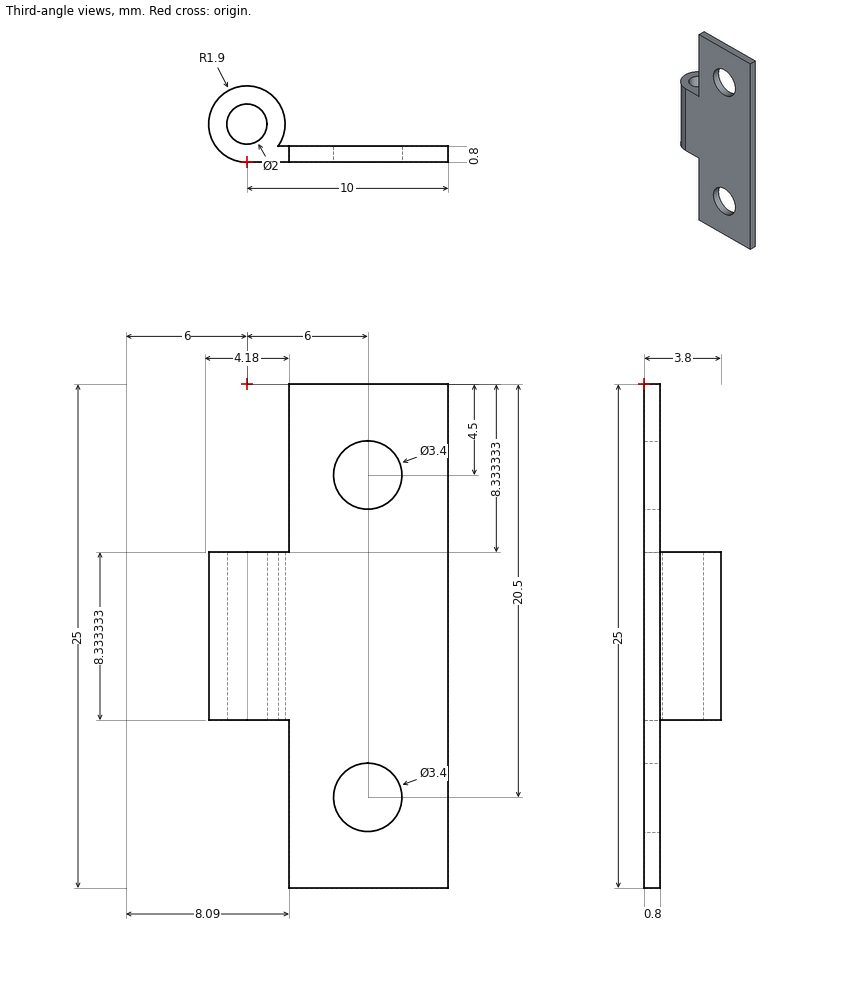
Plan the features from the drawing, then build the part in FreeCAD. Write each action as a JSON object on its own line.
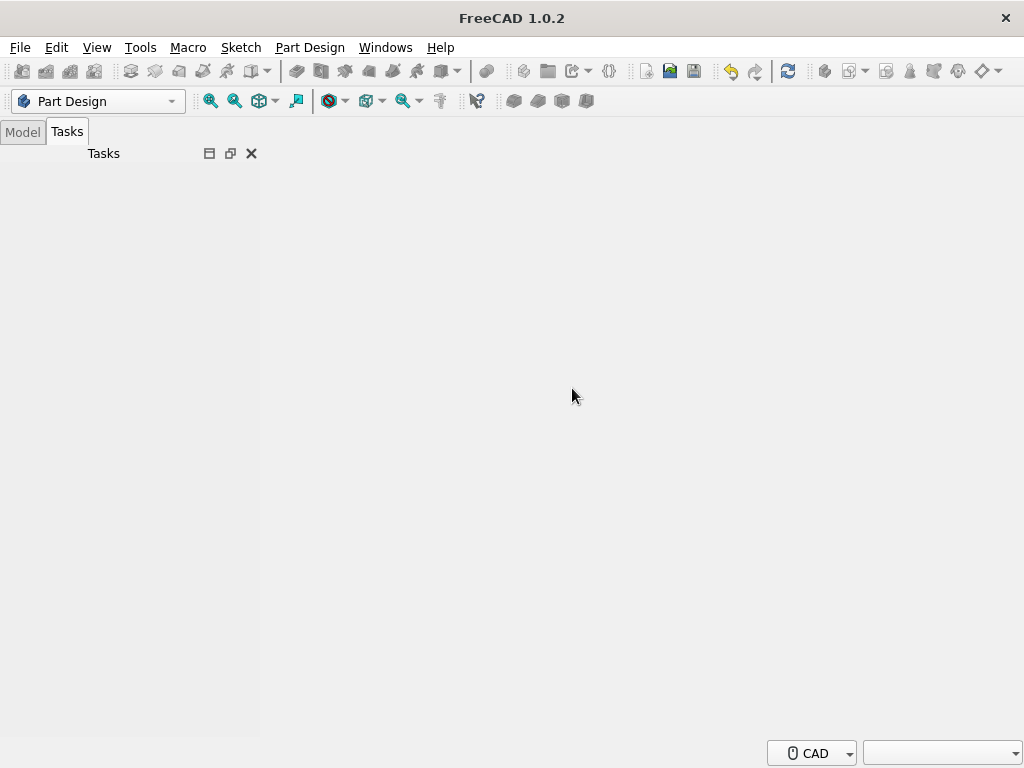
{"action": "left_click", "coordinate": [646, 72]}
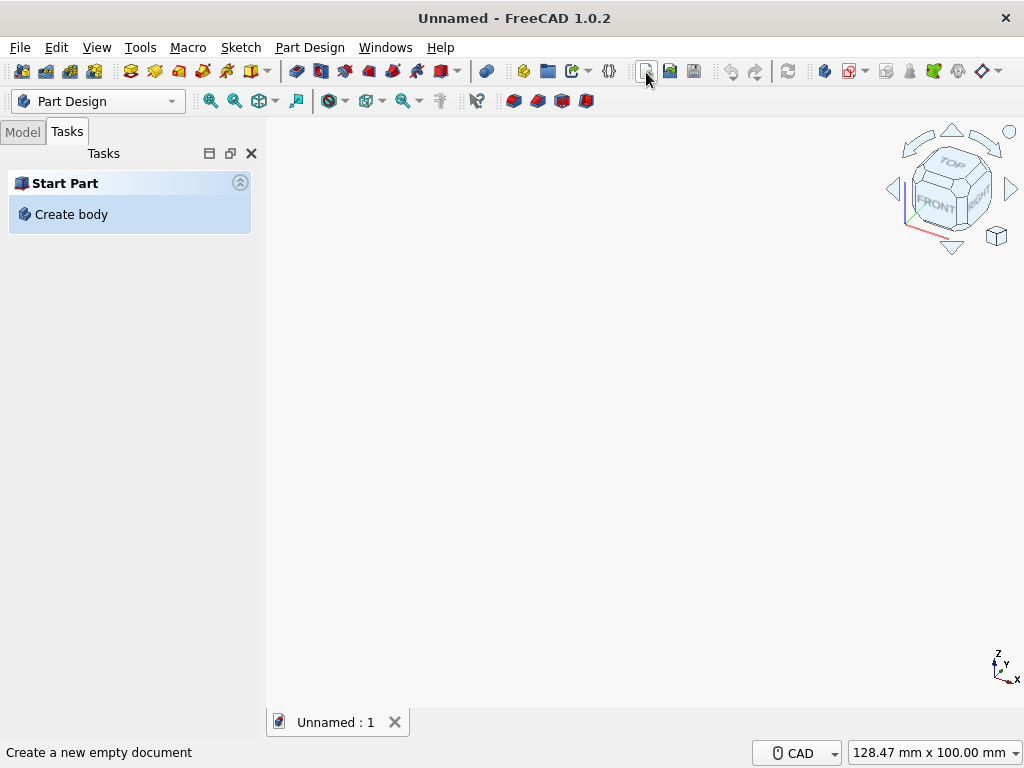
{"action": "left_click", "coordinate": [850, 72]}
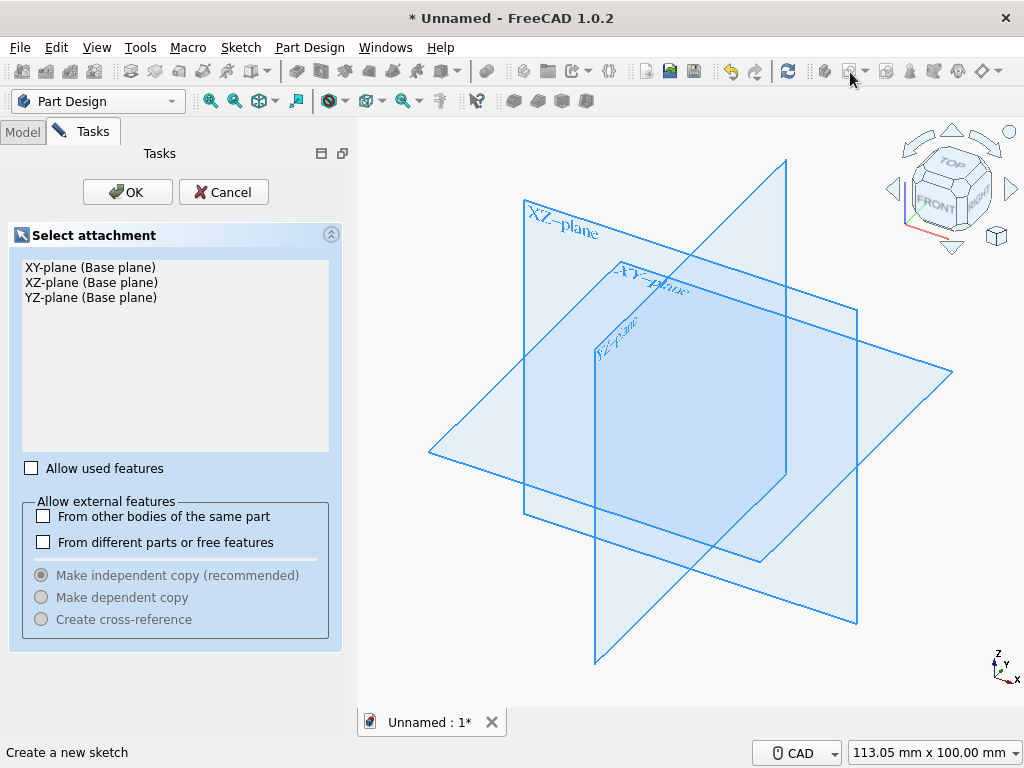
{"action": "left_click", "coordinate": [82, 268]}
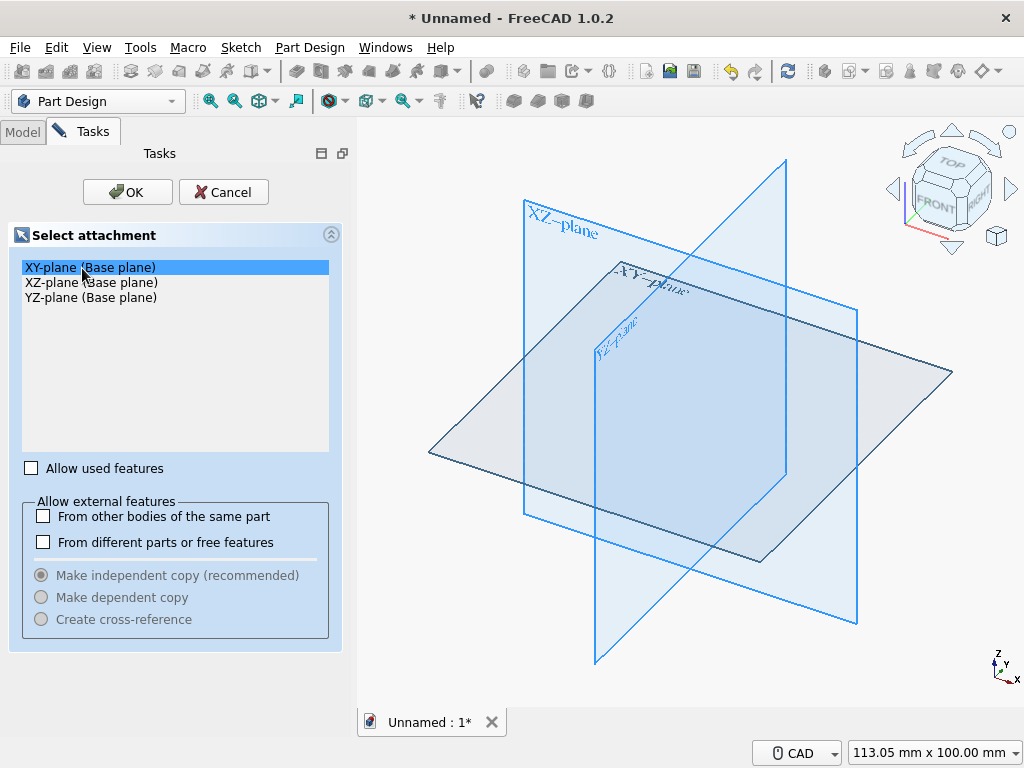
{"action": "left_click", "coordinate": [128, 192]}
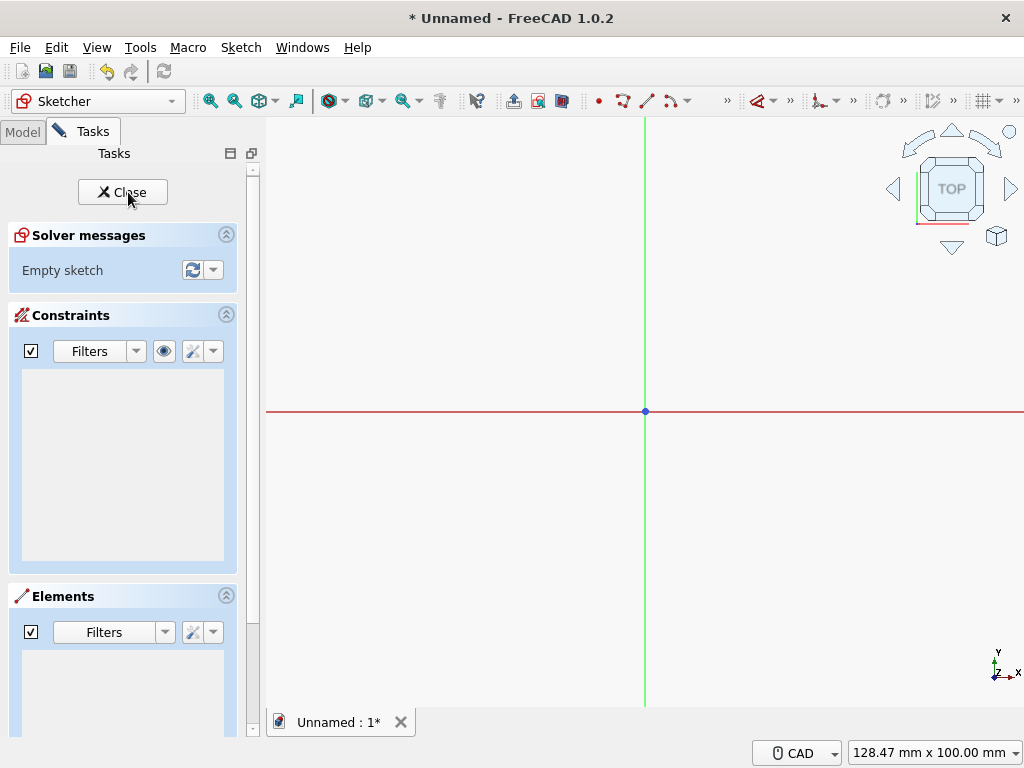
{"action": "scroll", "coordinate": [690, 399], "scroll_direction": "up", "scroll_amount": 9}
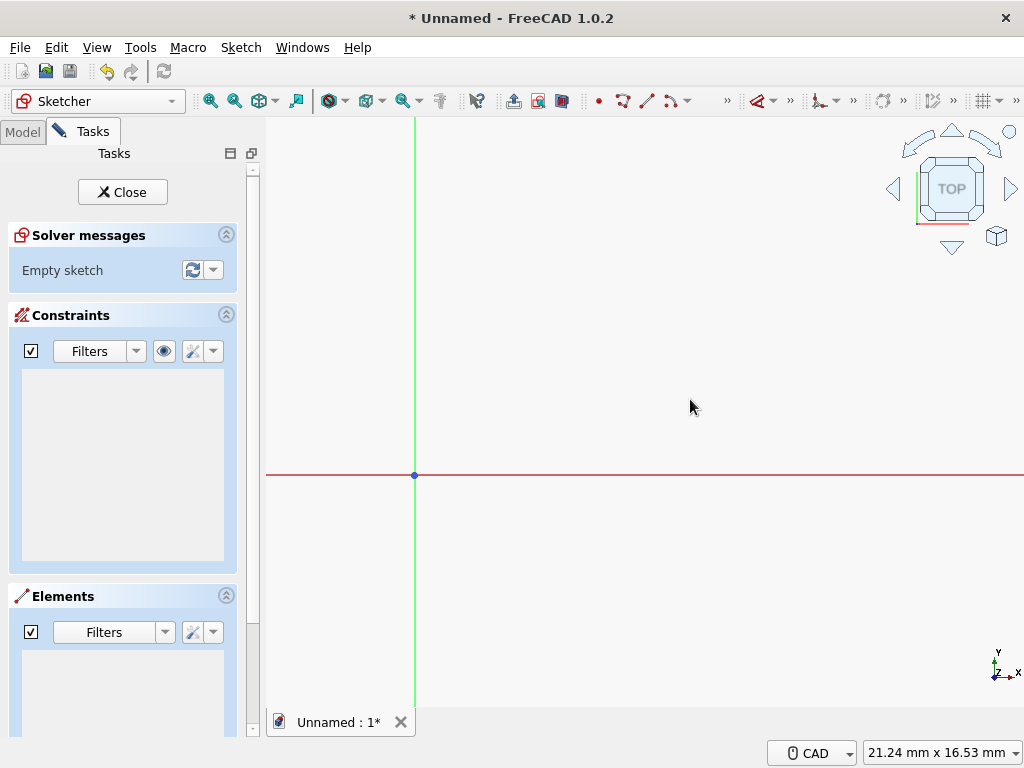
{"action": "left_click", "coordinate": [624, 102]}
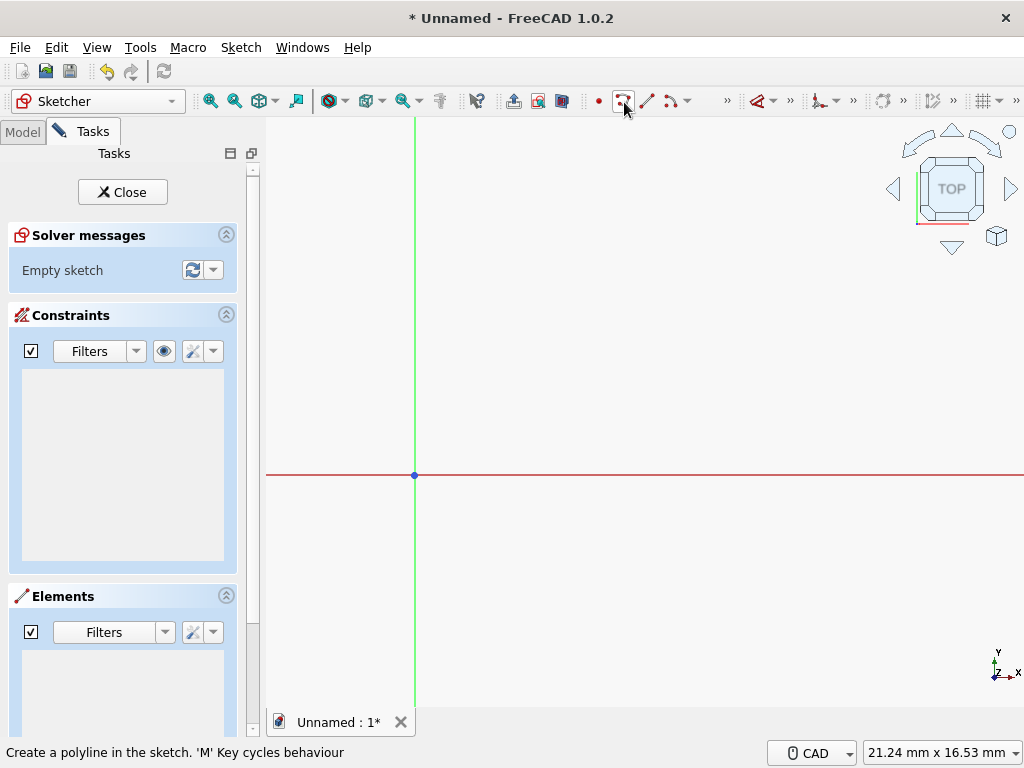
{"action": "left_click", "coordinate": [415, 475]}
{"action": "left_click", "coordinate": [772, 466]}
{"action": "left_click", "coordinate": [772, 447]}
{"action": "left_click", "coordinate": [470, 447]}
{"action": "right_click", "coordinate": [470, 447]}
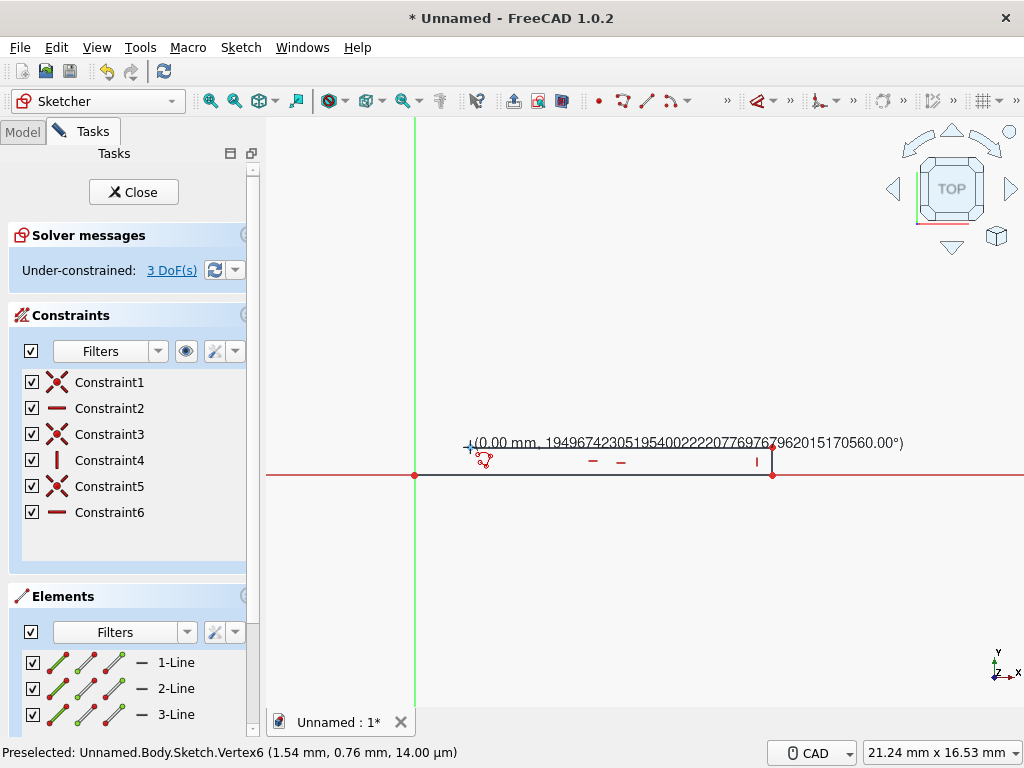
{"action": "left_click", "coordinate": [690, 102]}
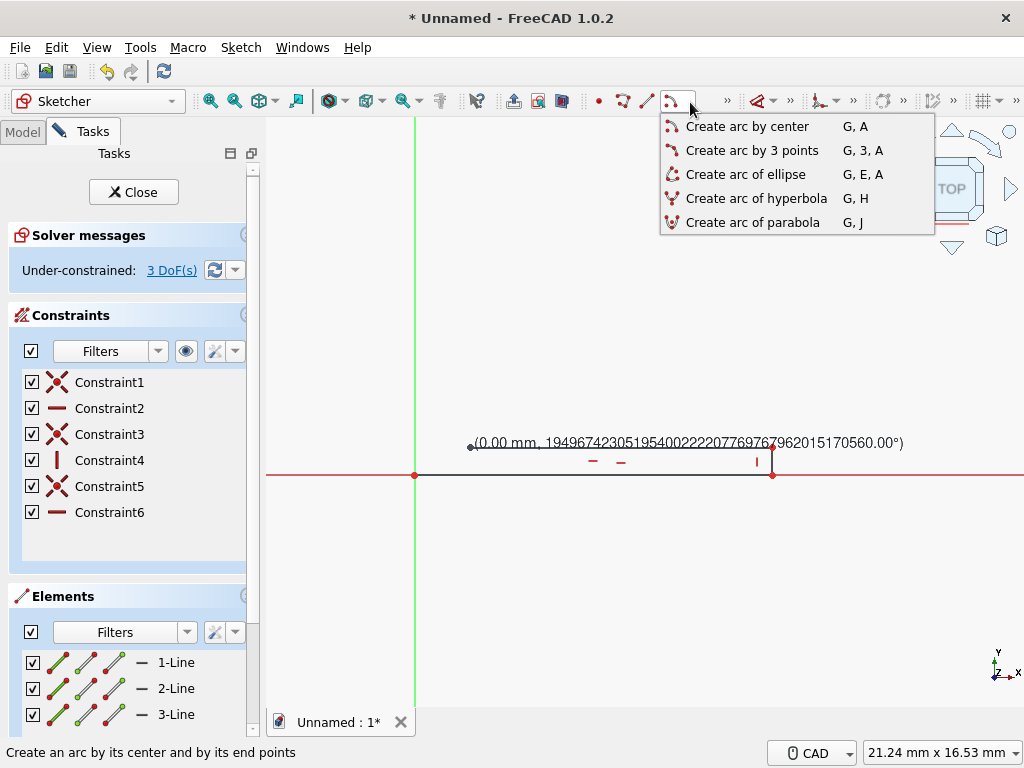
{"action": "left_click", "coordinate": [798, 150]}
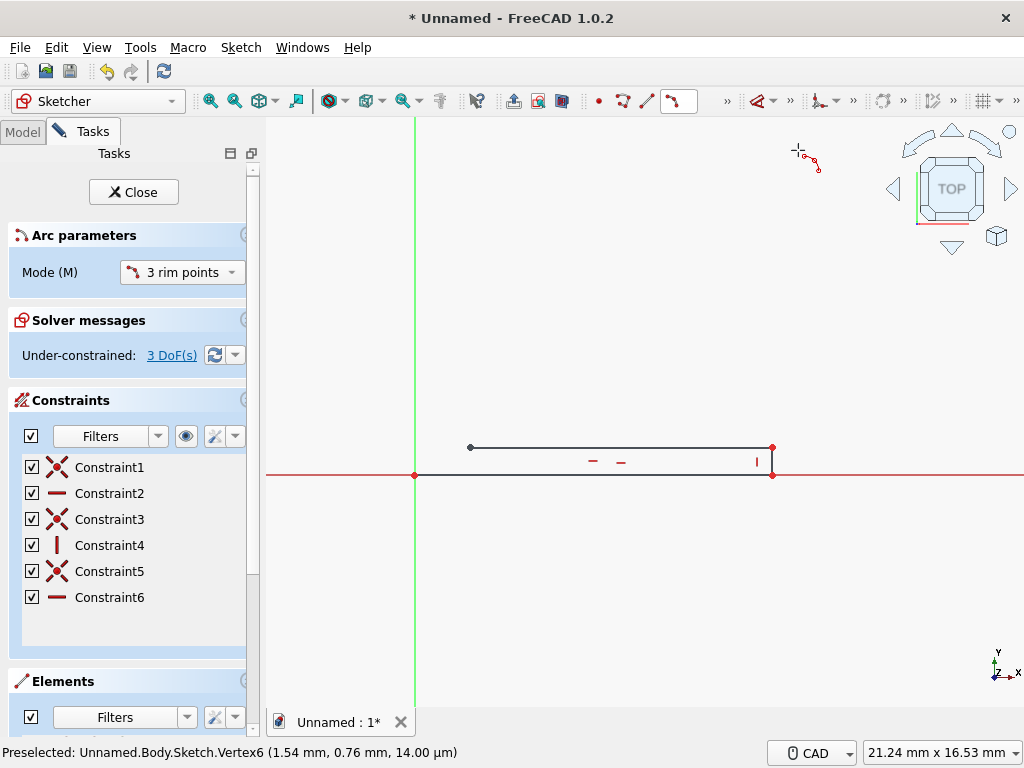
{"action": "left_click", "coordinate": [470, 448]}
{"action": "left_click", "coordinate": [415, 475]}
{"action": "left_click", "coordinate": [384, 347]}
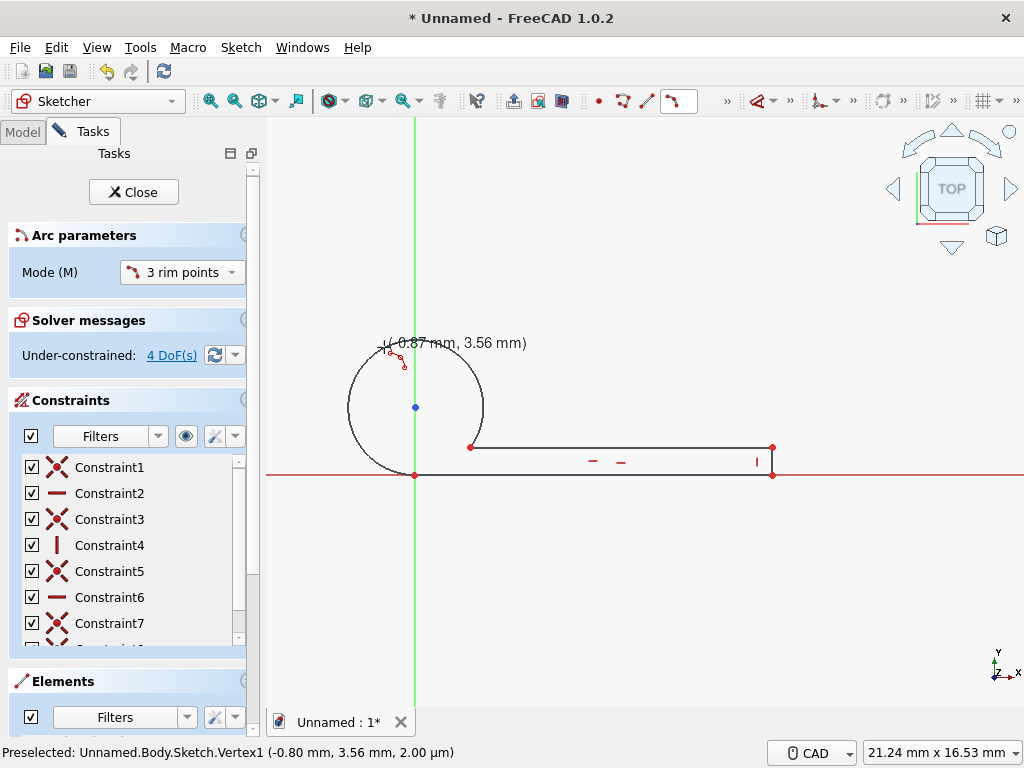
{"action": "key", "text": "g c"}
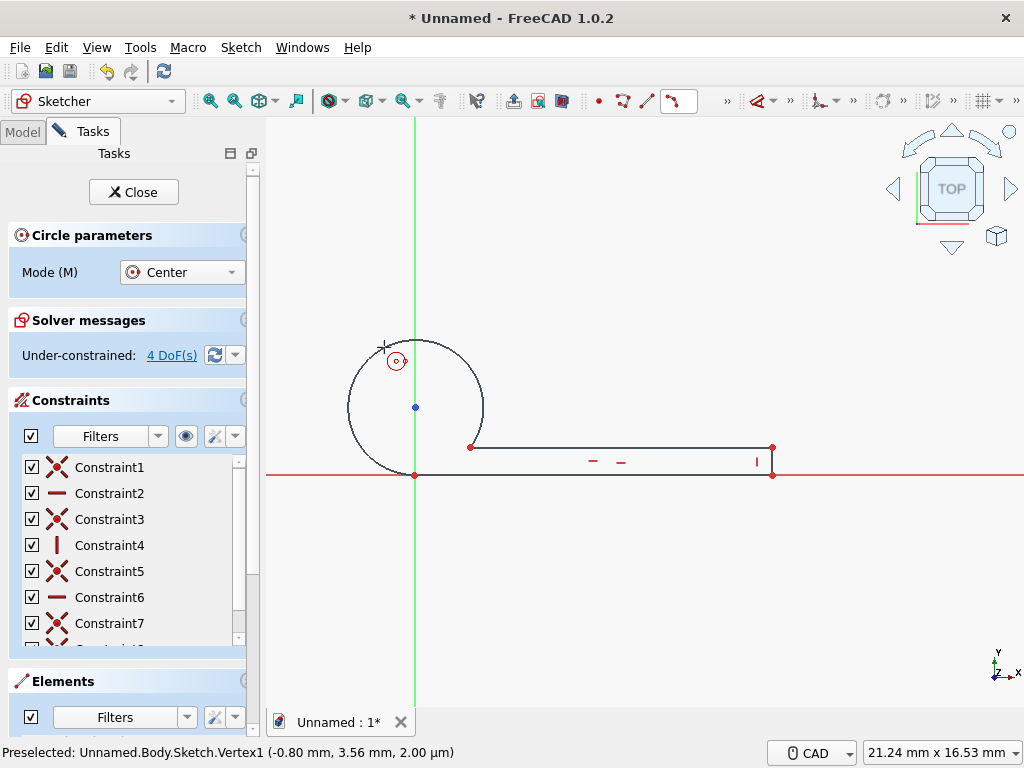
{"action": "left_click", "coordinate": [415, 407]}
{"action": "left_click", "coordinate": [440, 382]}
{"action": "key", "text": "Escape"}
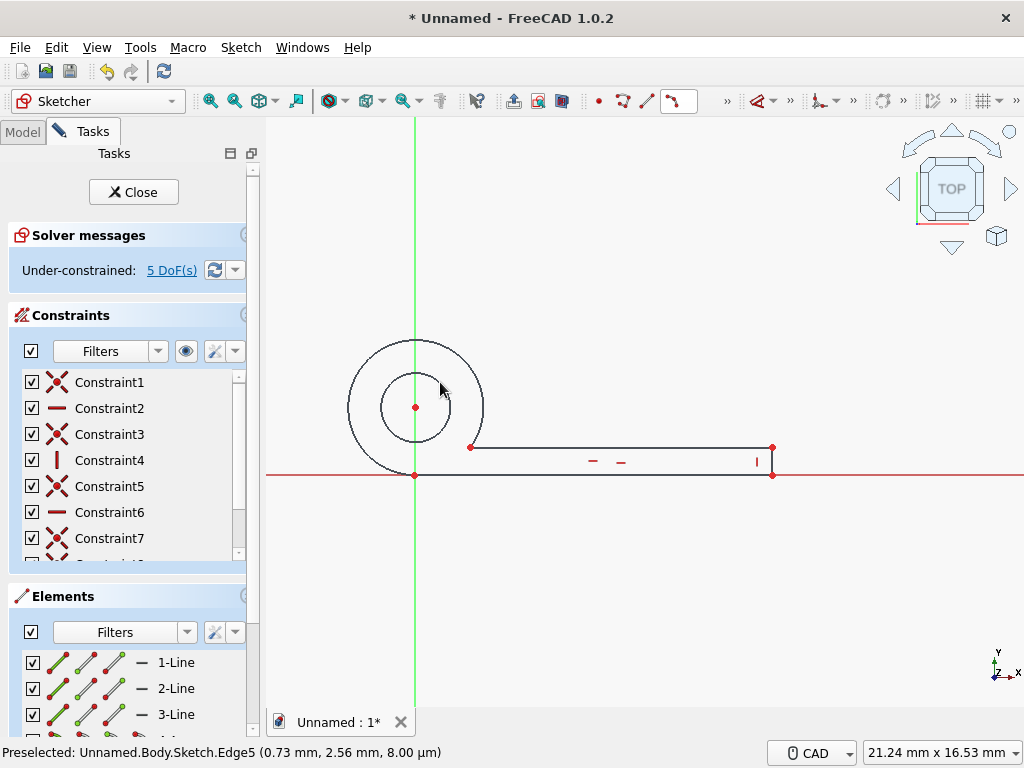
{"action": "left_click", "coordinate": [522, 475]}